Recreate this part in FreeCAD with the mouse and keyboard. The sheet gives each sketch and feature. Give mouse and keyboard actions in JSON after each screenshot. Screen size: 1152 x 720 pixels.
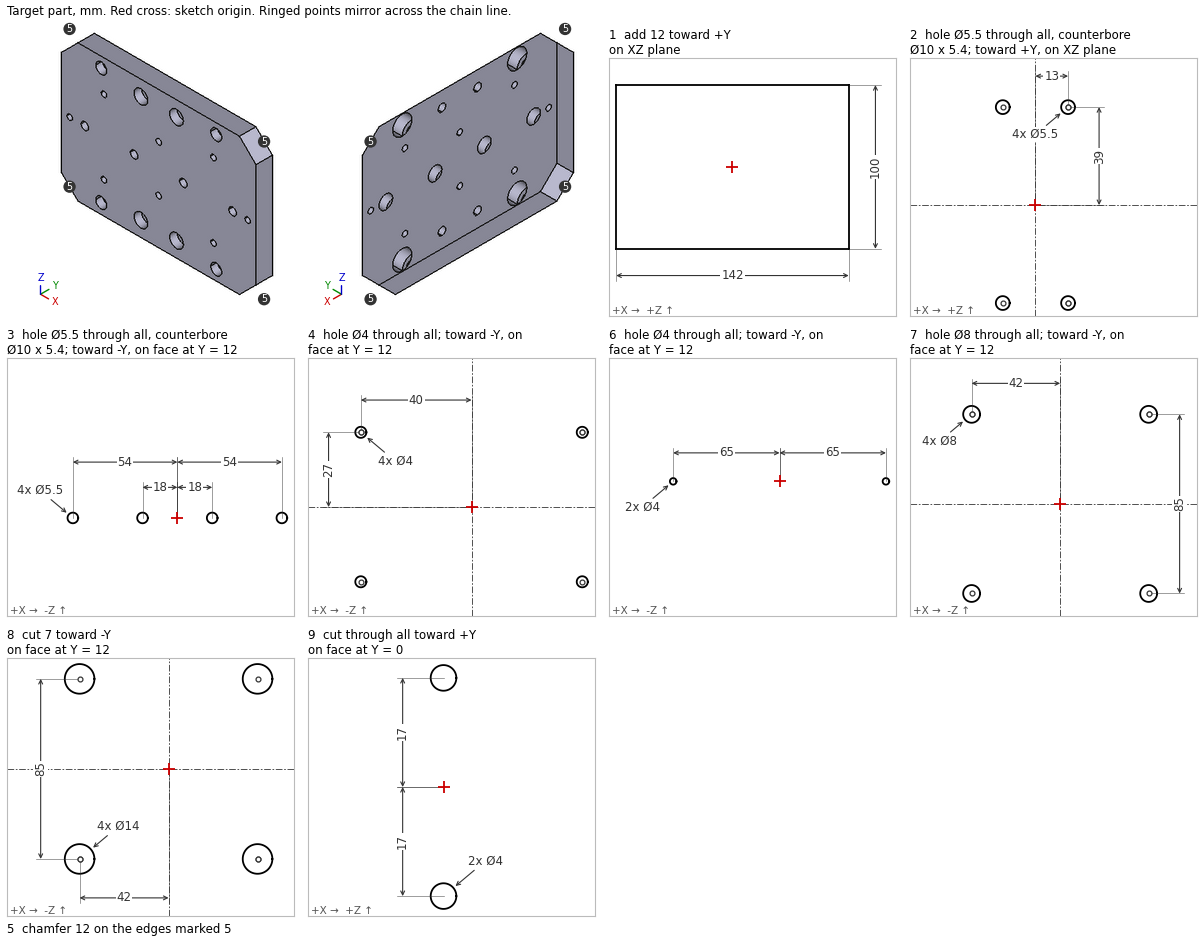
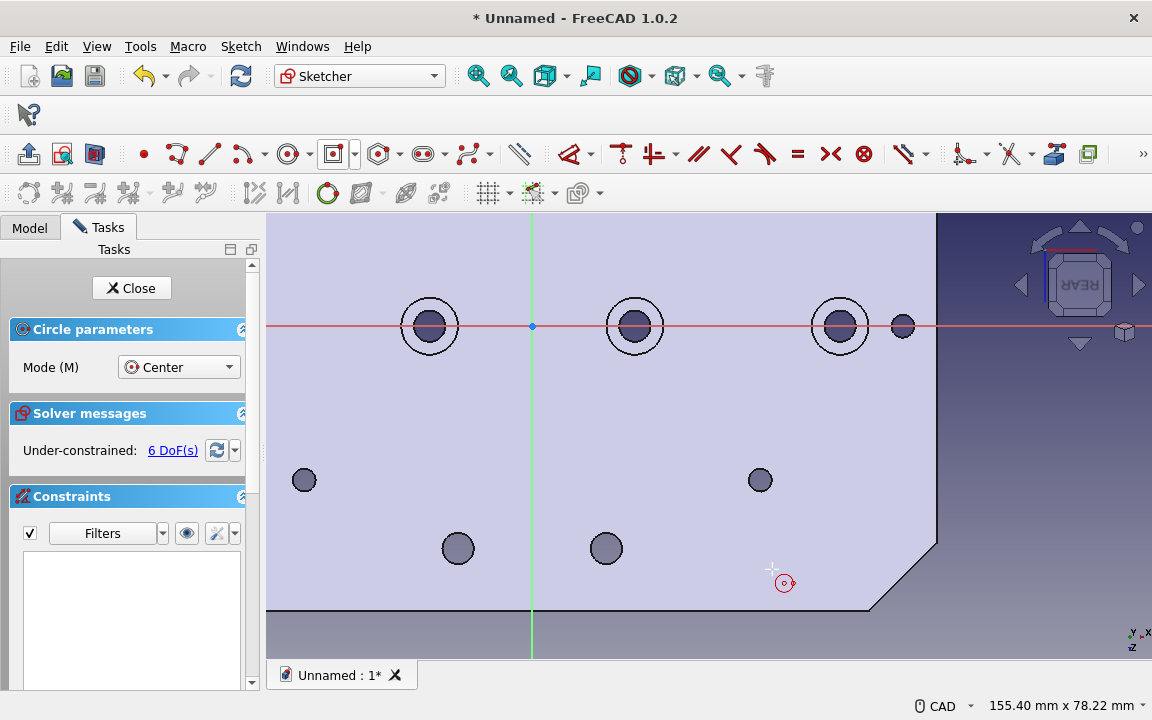
{"action": "left_click", "coordinate": [772, 569]}
{"action": "left_click", "coordinate": [788, 552]}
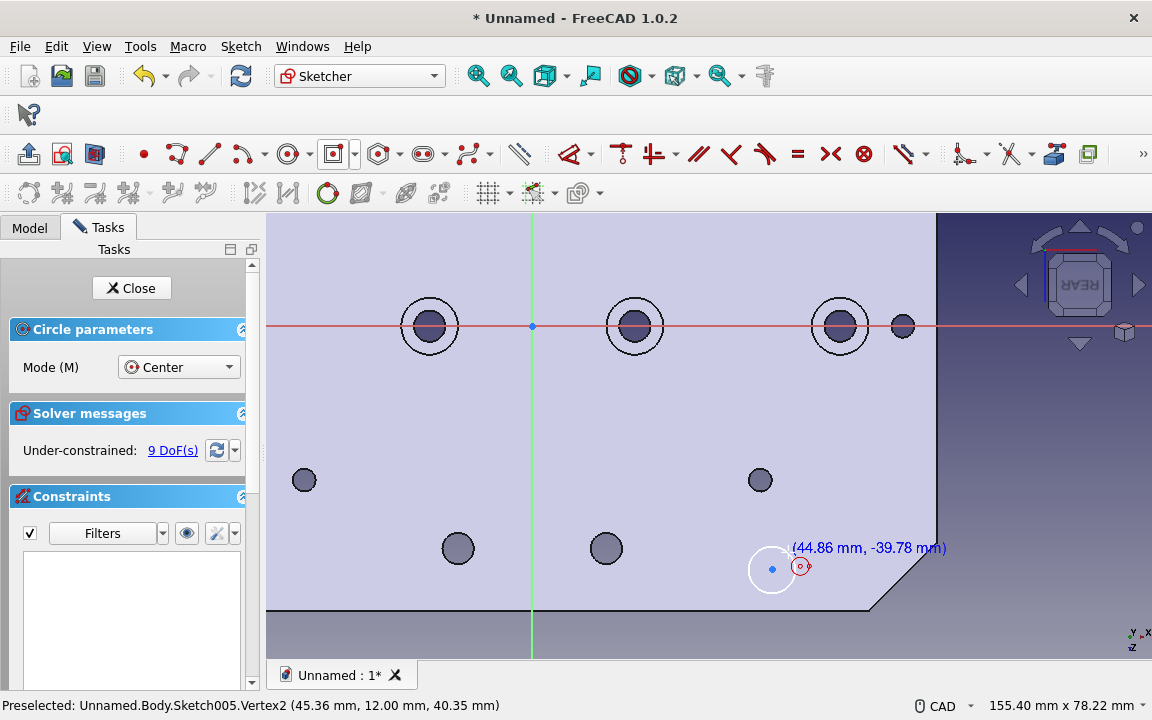
{"action": "scroll", "coordinate": [772, 570], "scroll_direction": "down", "scroll_amount": 3}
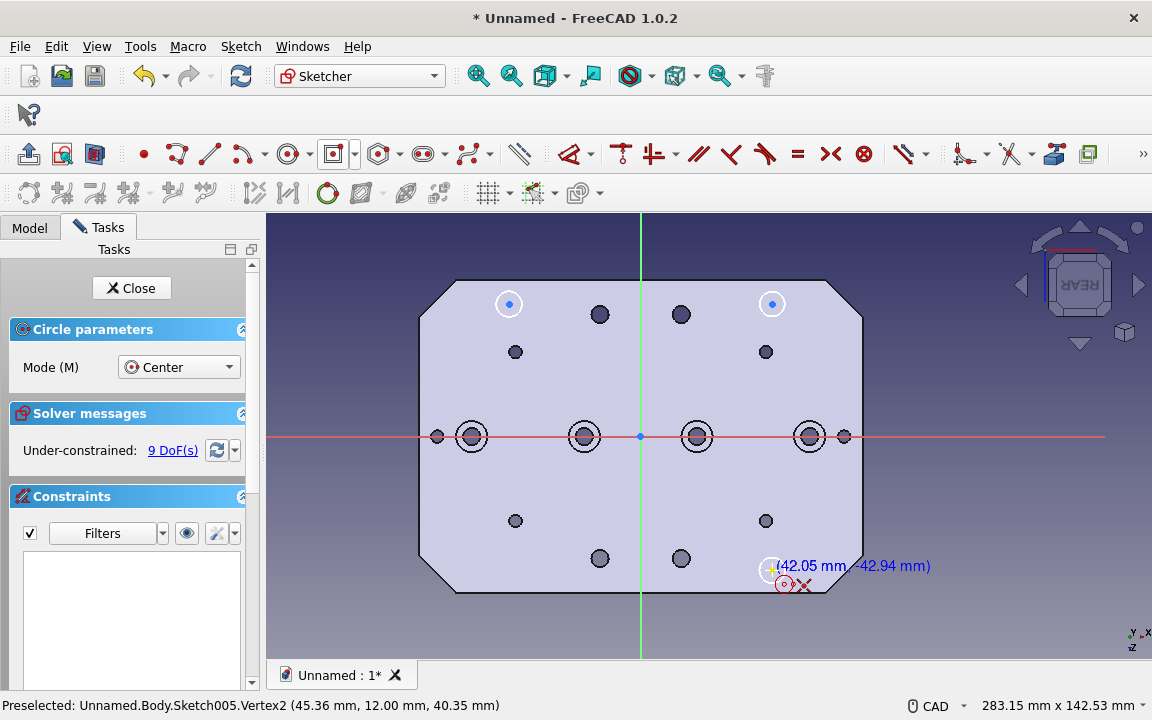
{"action": "scroll", "coordinate": [509, 570], "scroll_direction": "up", "scroll_amount": 3}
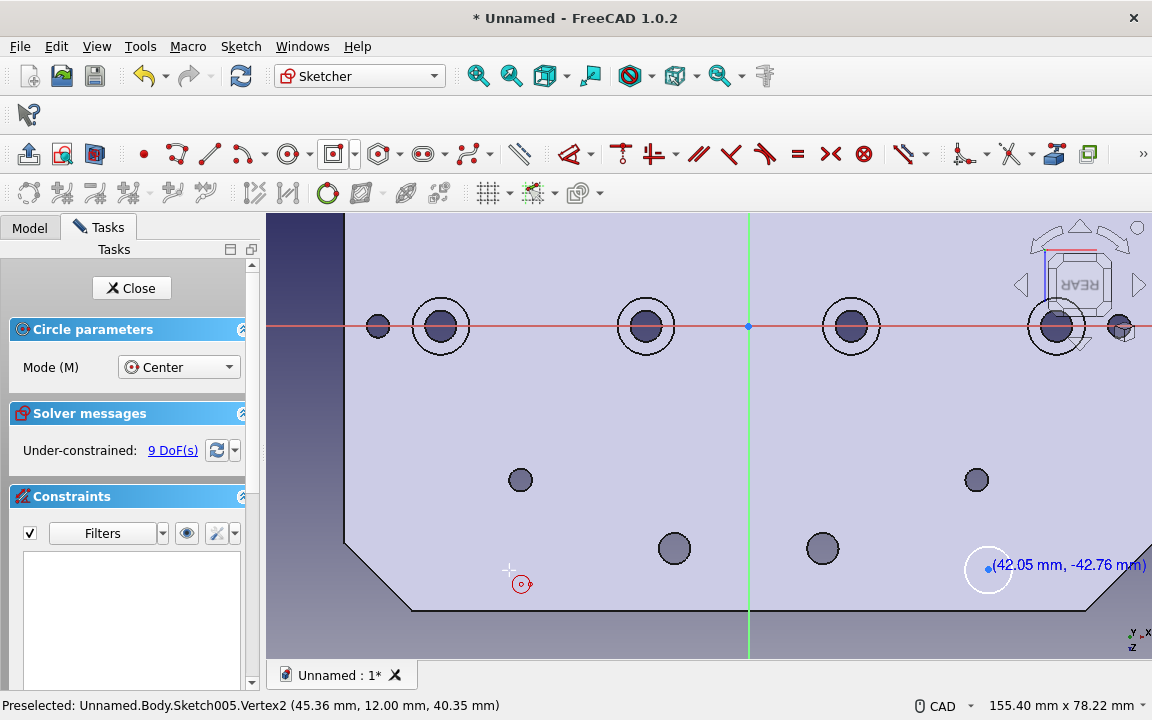
{"action": "left_click", "coordinate": [509, 569]}
{"action": "left_click", "coordinate": [525, 552]}
{"action": "key", "text": "Escape"}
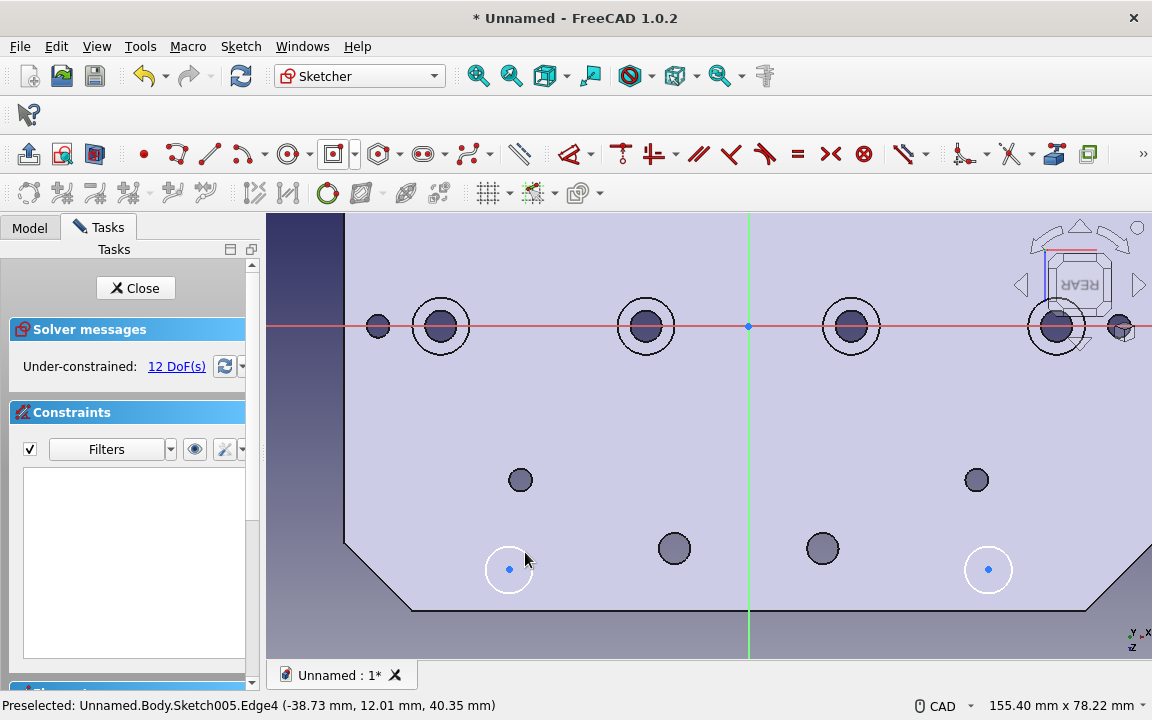
{"action": "scroll", "coordinate": [509, 570], "scroll_direction": "down", "scroll_amount": 3}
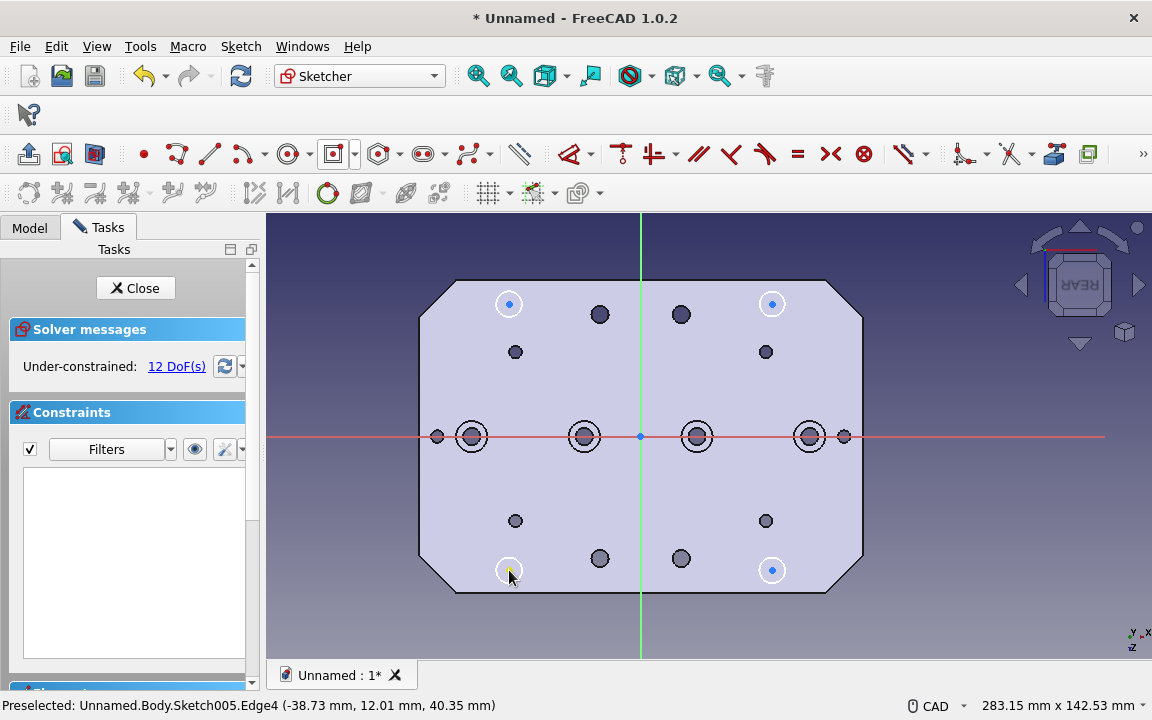
{"action": "left_click", "coordinate": [518, 295]}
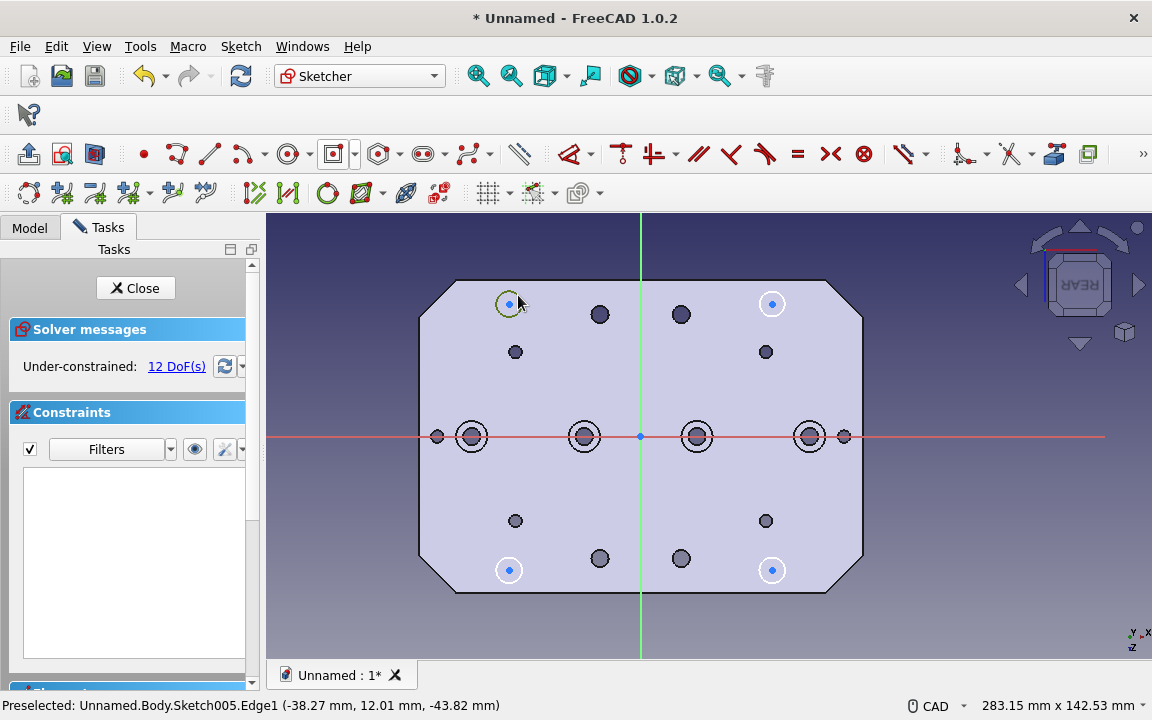
{"action": "left_click", "coordinate": [781, 295]}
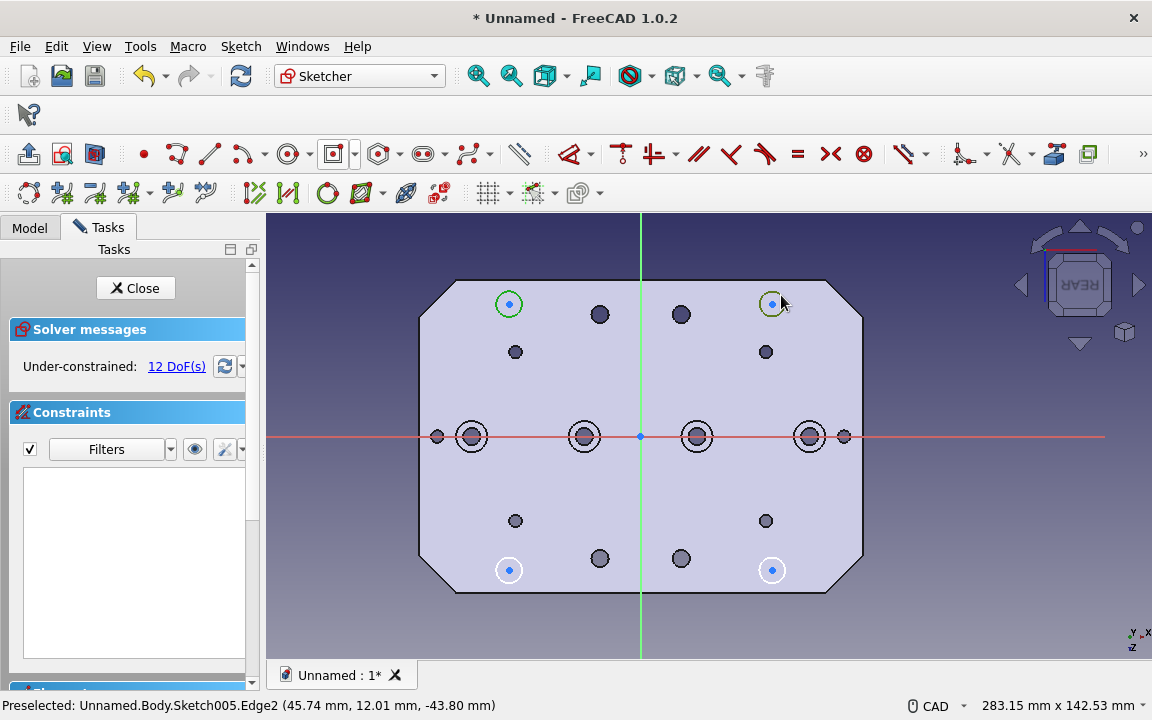
{"action": "left_click", "coordinate": [781, 561]}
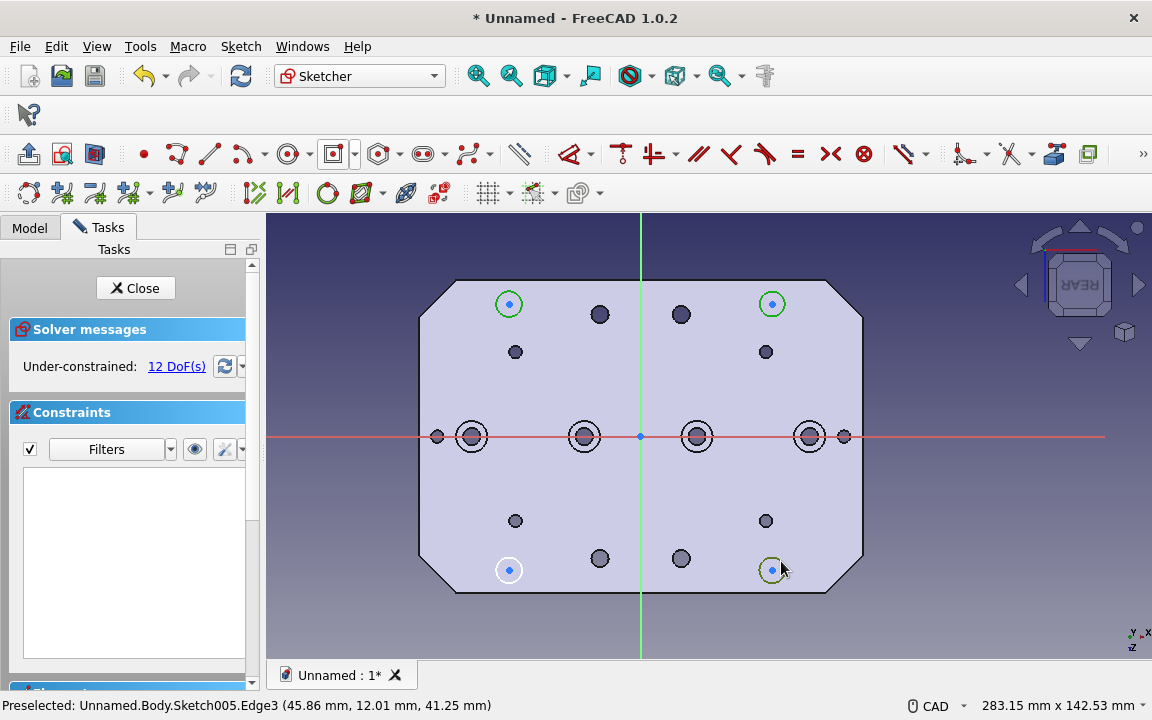
{"action": "left_click", "coordinate": [518, 561]}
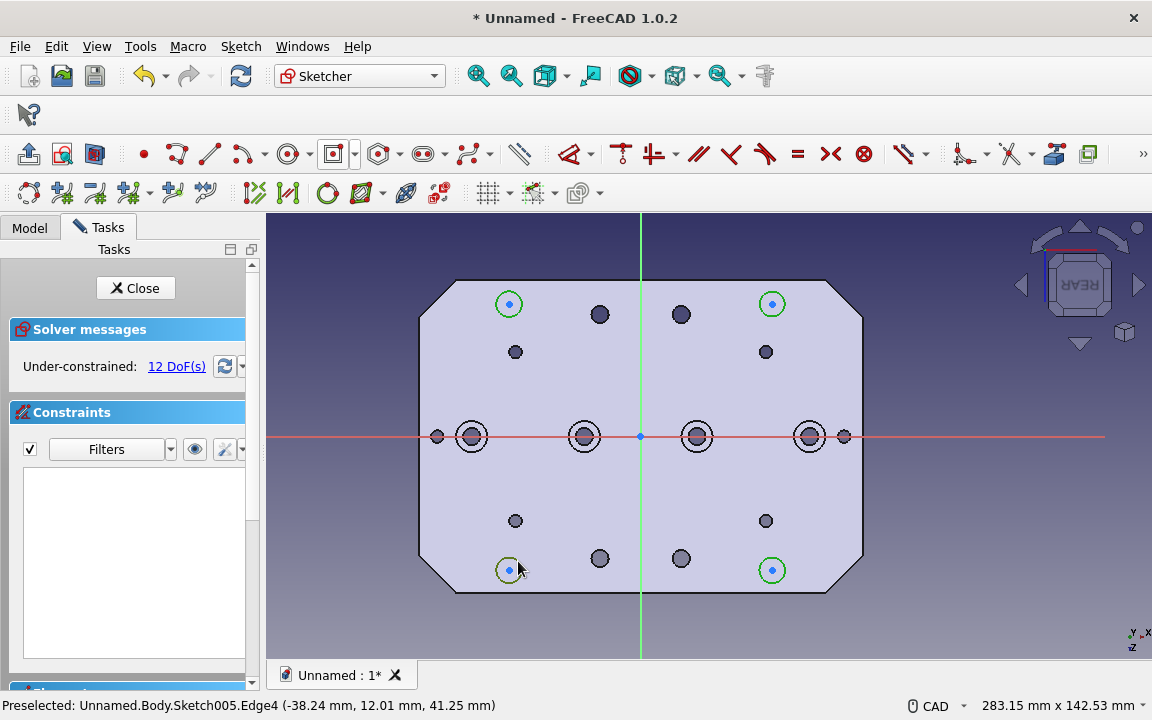
{"action": "left_click", "coordinate": [798, 154]}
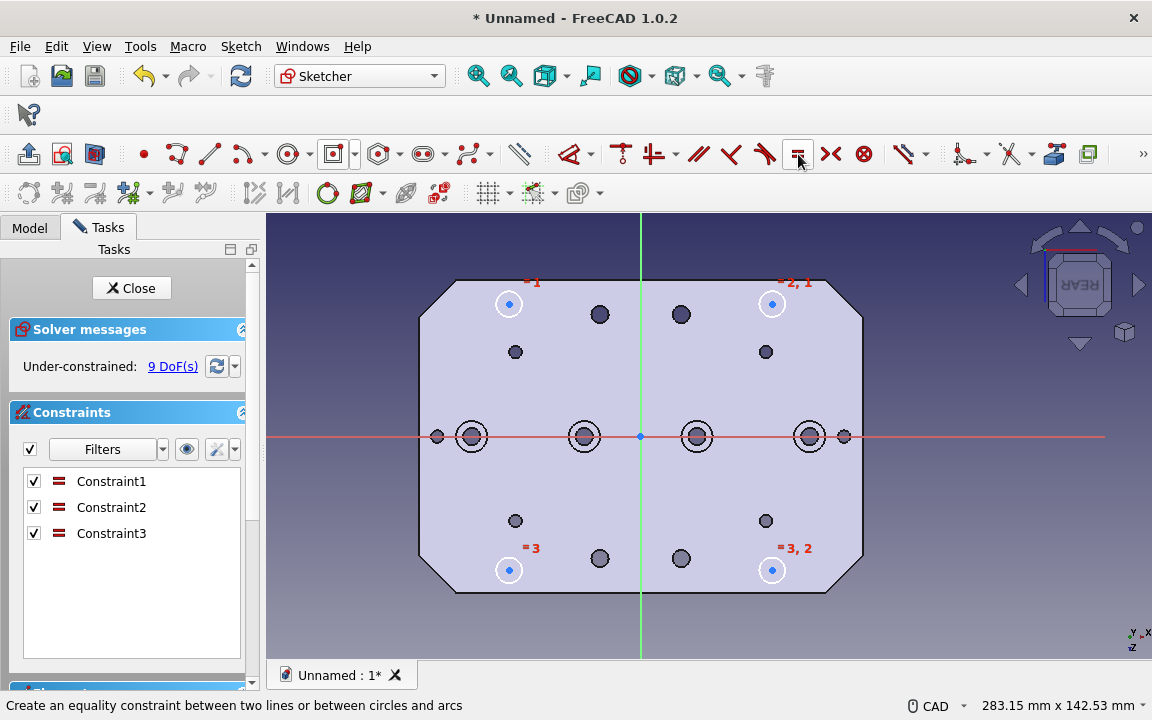
{"action": "left_click", "coordinate": [509, 304]}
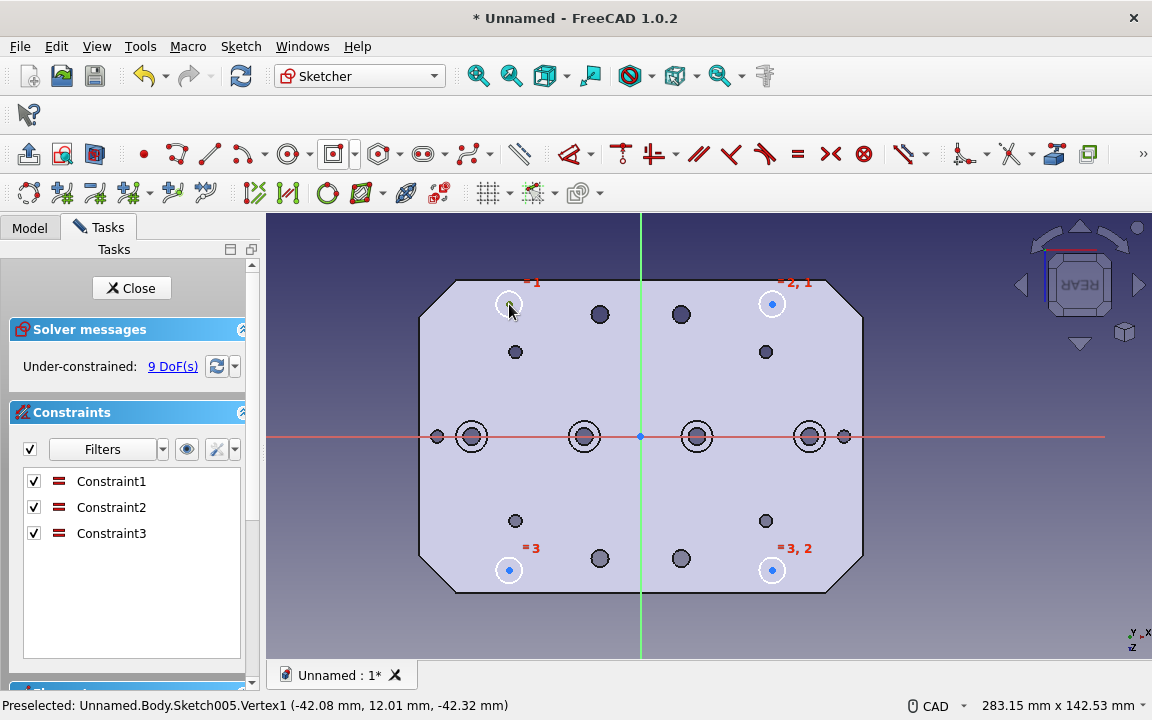
{"action": "left_click", "coordinate": [772, 304]}